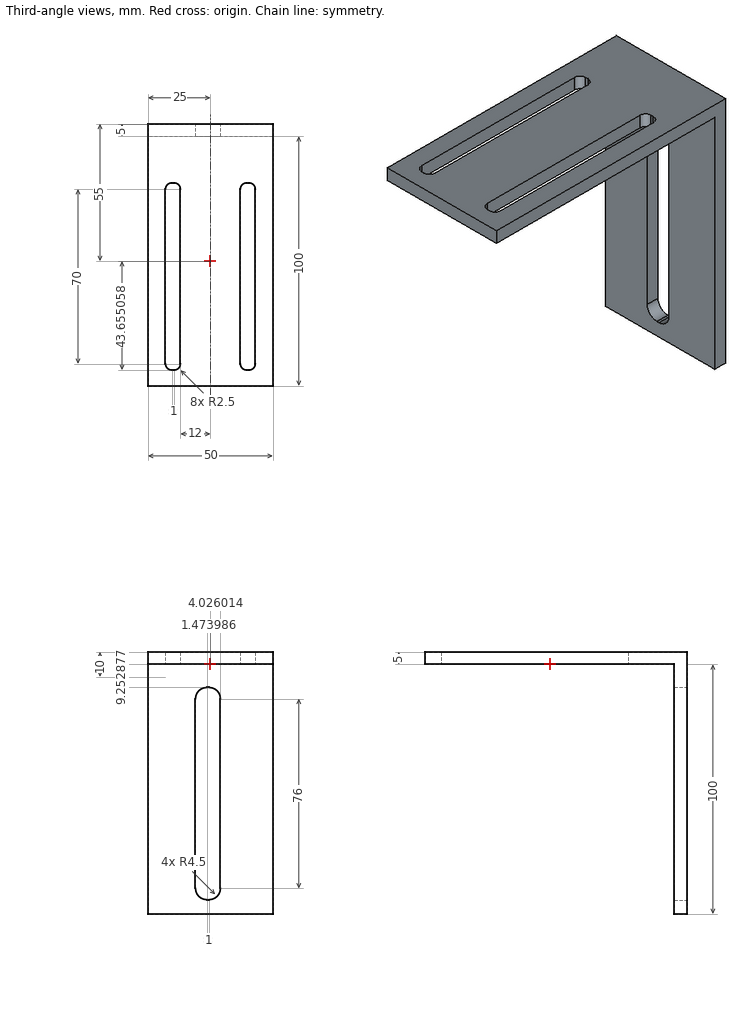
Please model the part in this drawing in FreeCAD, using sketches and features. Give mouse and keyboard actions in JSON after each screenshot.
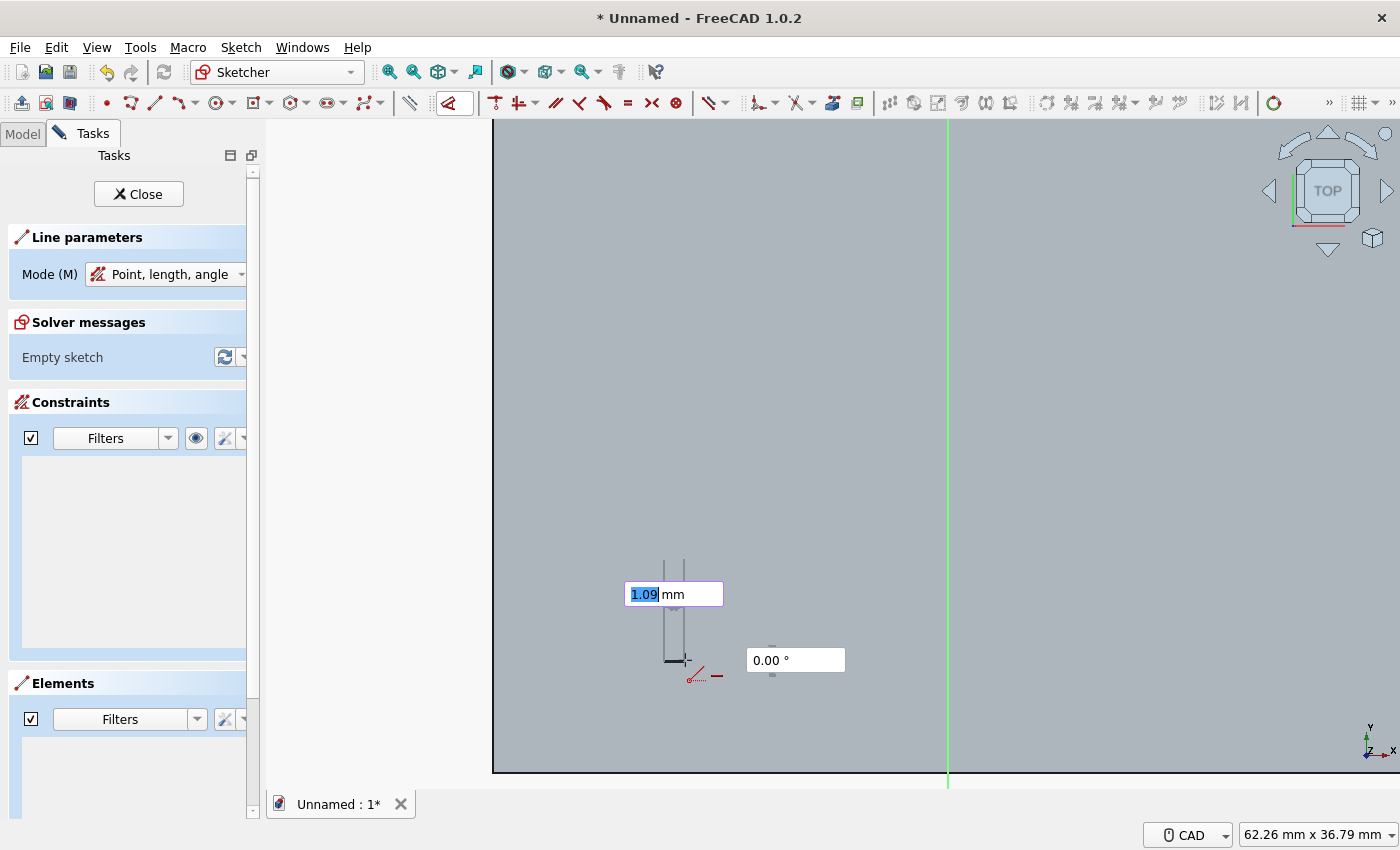
{"action": "left_click", "coordinate": [684, 658]}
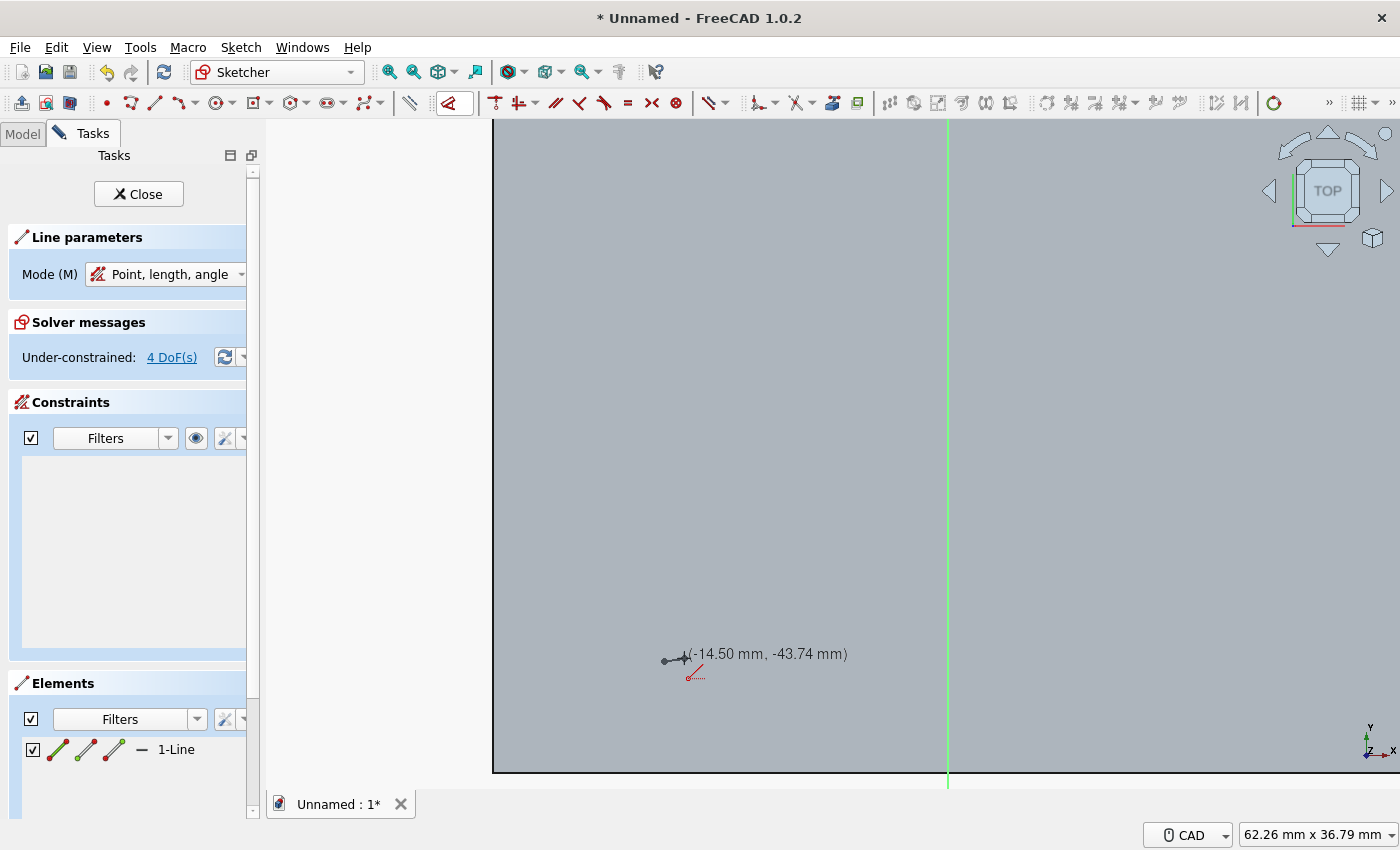
{"action": "left_click", "coordinate": [730, 612]}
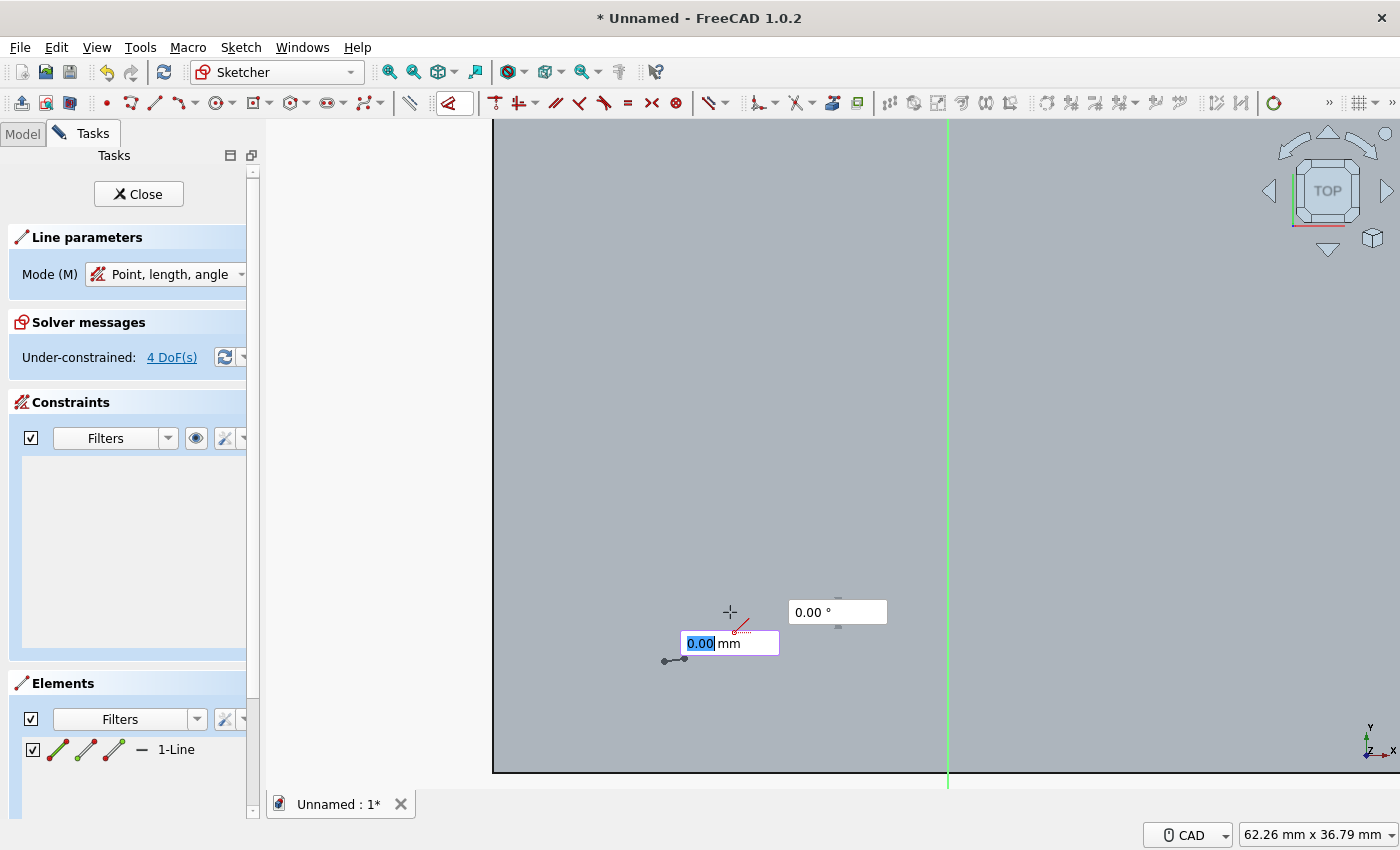
{"action": "scroll", "coordinate": [685, 661], "scroll_direction": "down", "scroll_amount": 6}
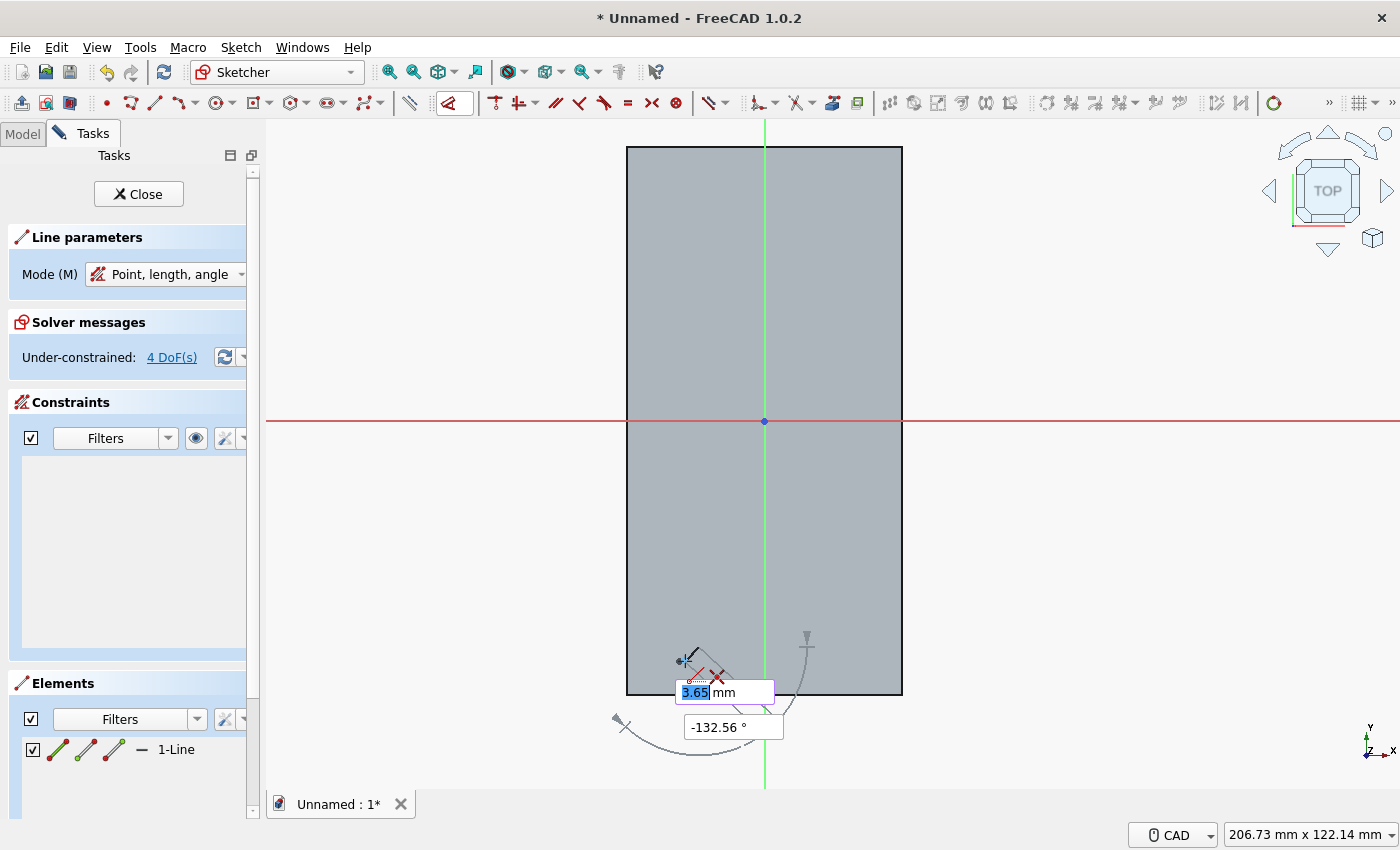
{"action": "left_click", "coordinate": [699, 263]}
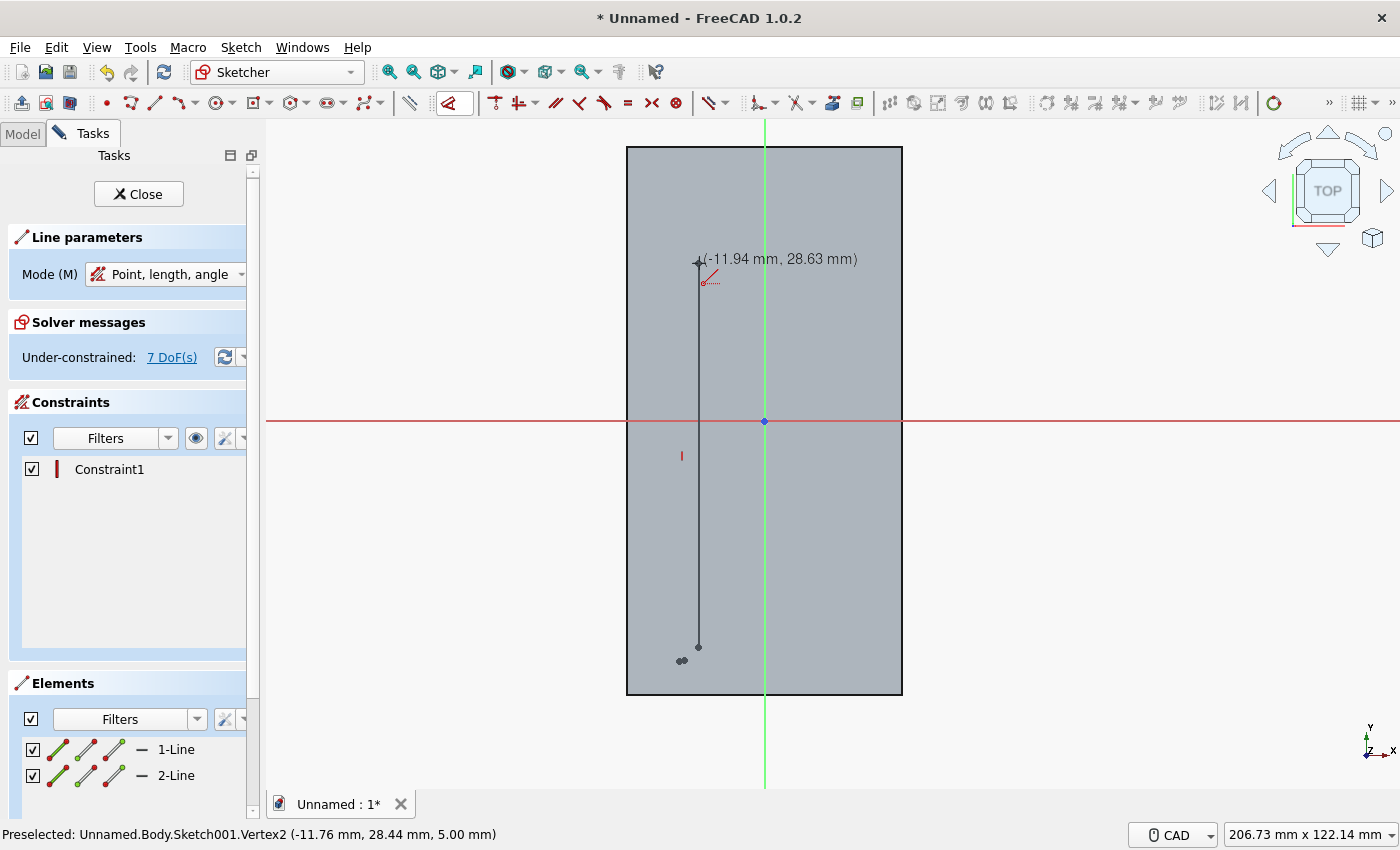
{"action": "left_click", "coordinate": [685, 249]}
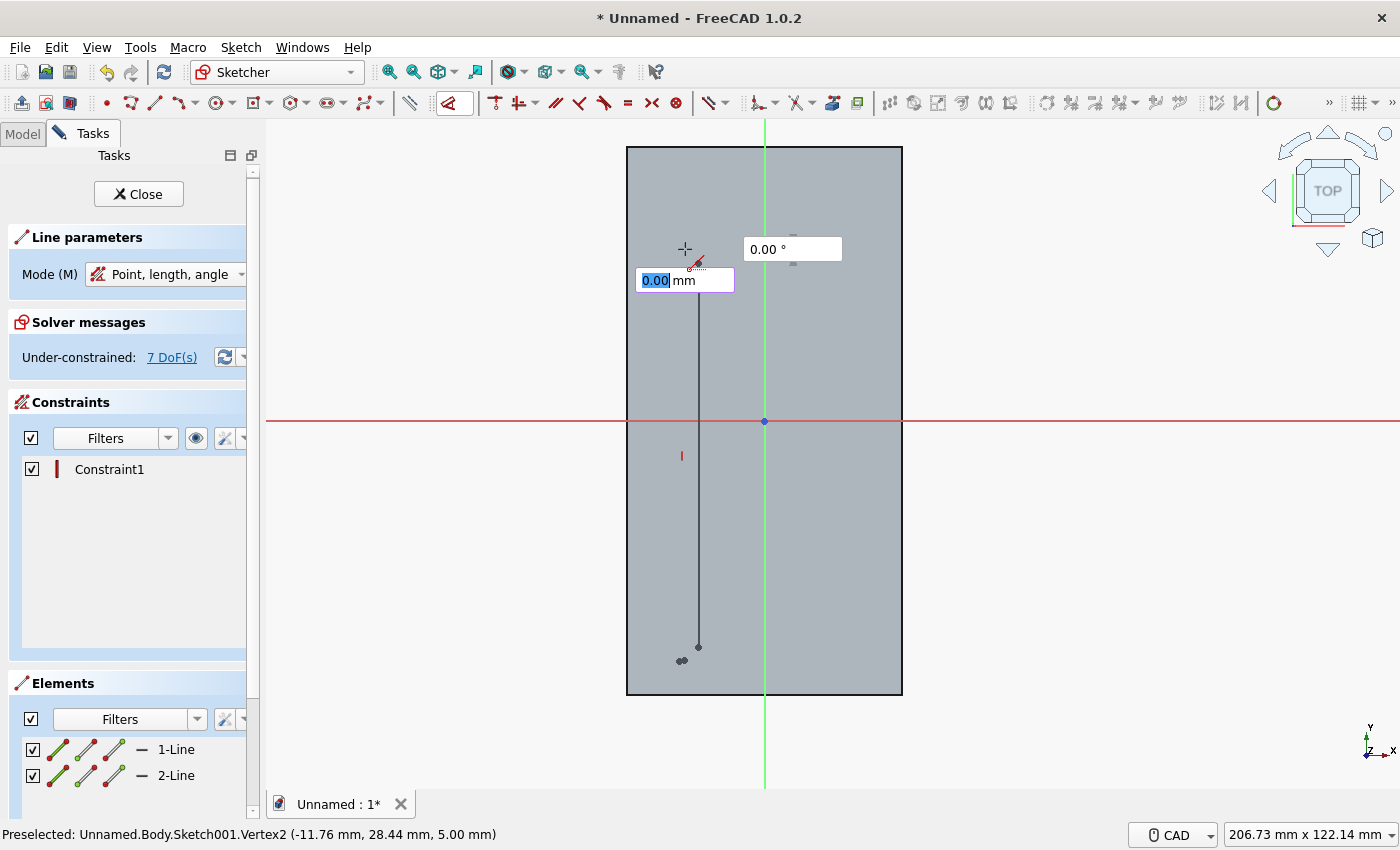
{"action": "scroll", "coordinate": [679, 249], "scroll_direction": "up", "scroll_amount": 6}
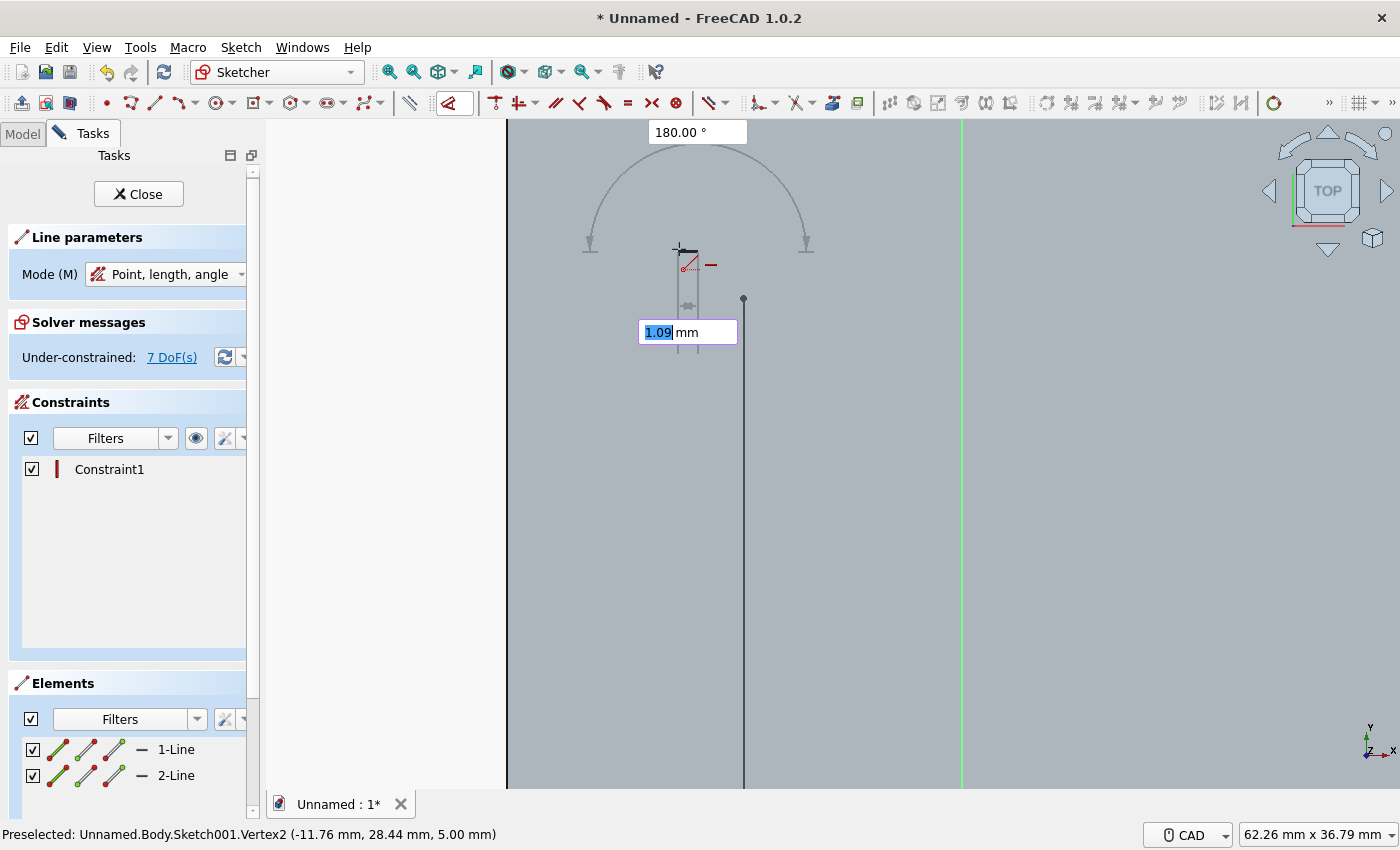
{"action": "left_click", "coordinate": [680, 249]}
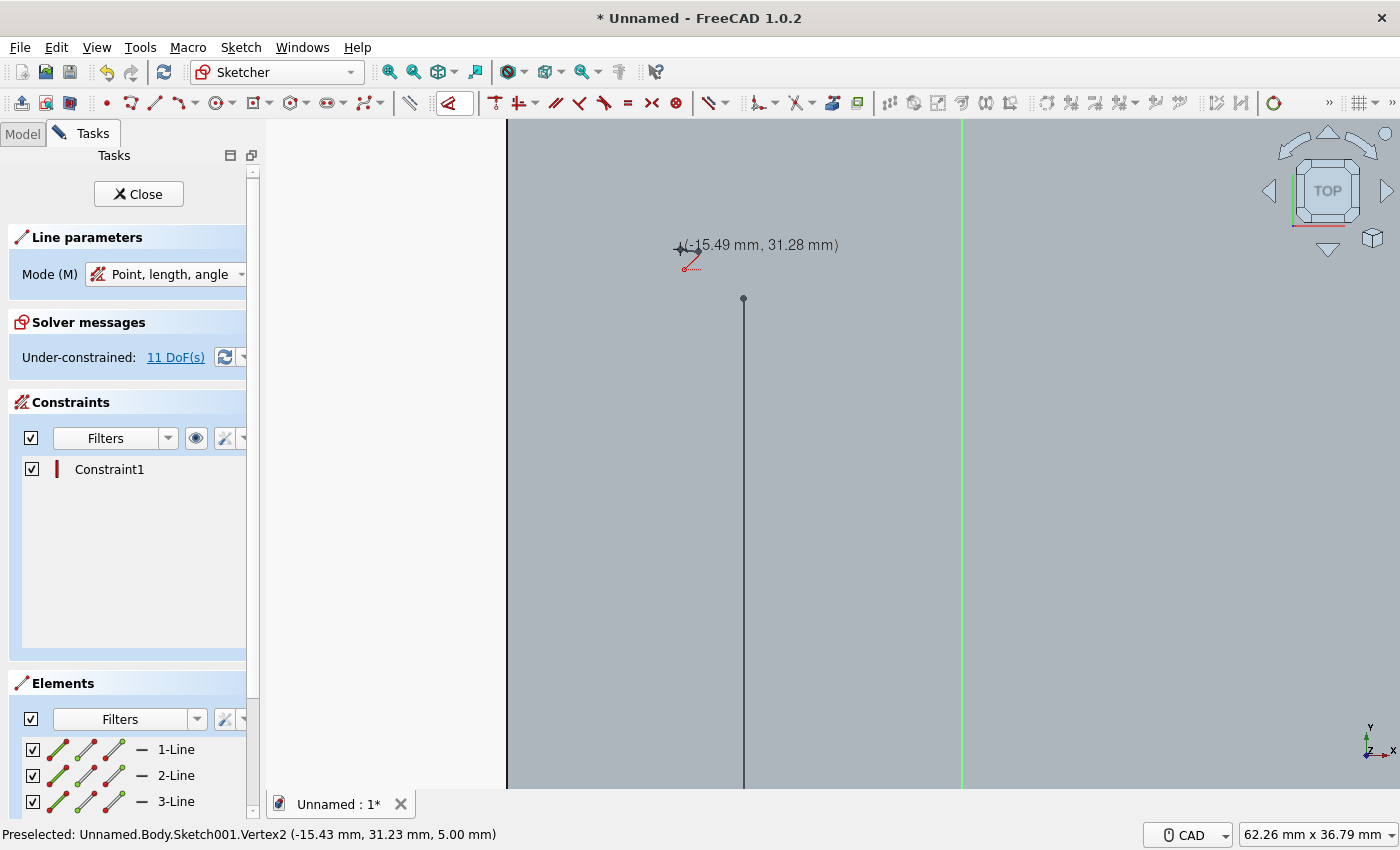
{"action": "left_click", "coordinate": [634, 294]}